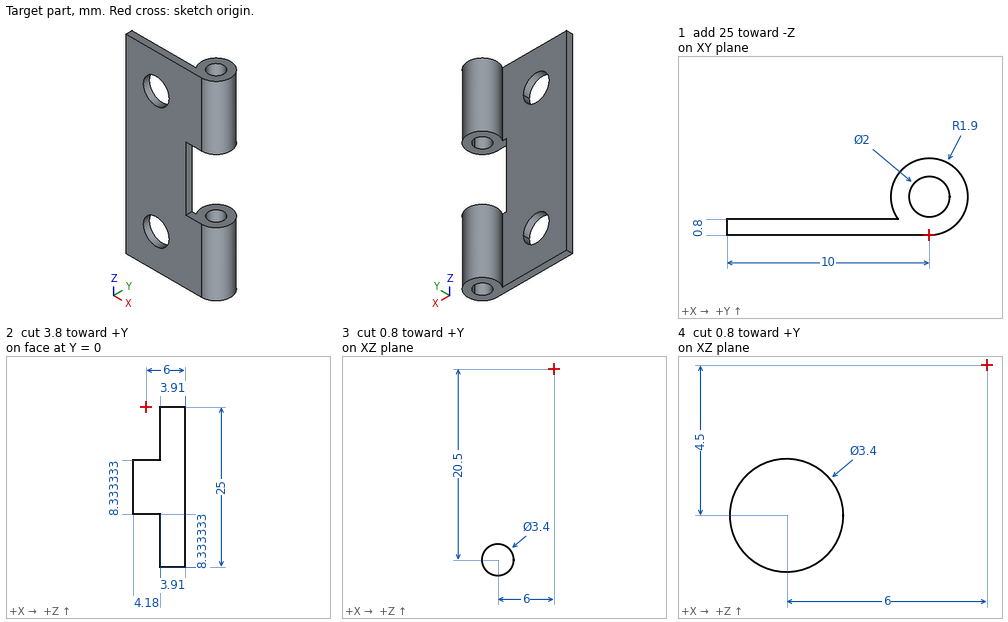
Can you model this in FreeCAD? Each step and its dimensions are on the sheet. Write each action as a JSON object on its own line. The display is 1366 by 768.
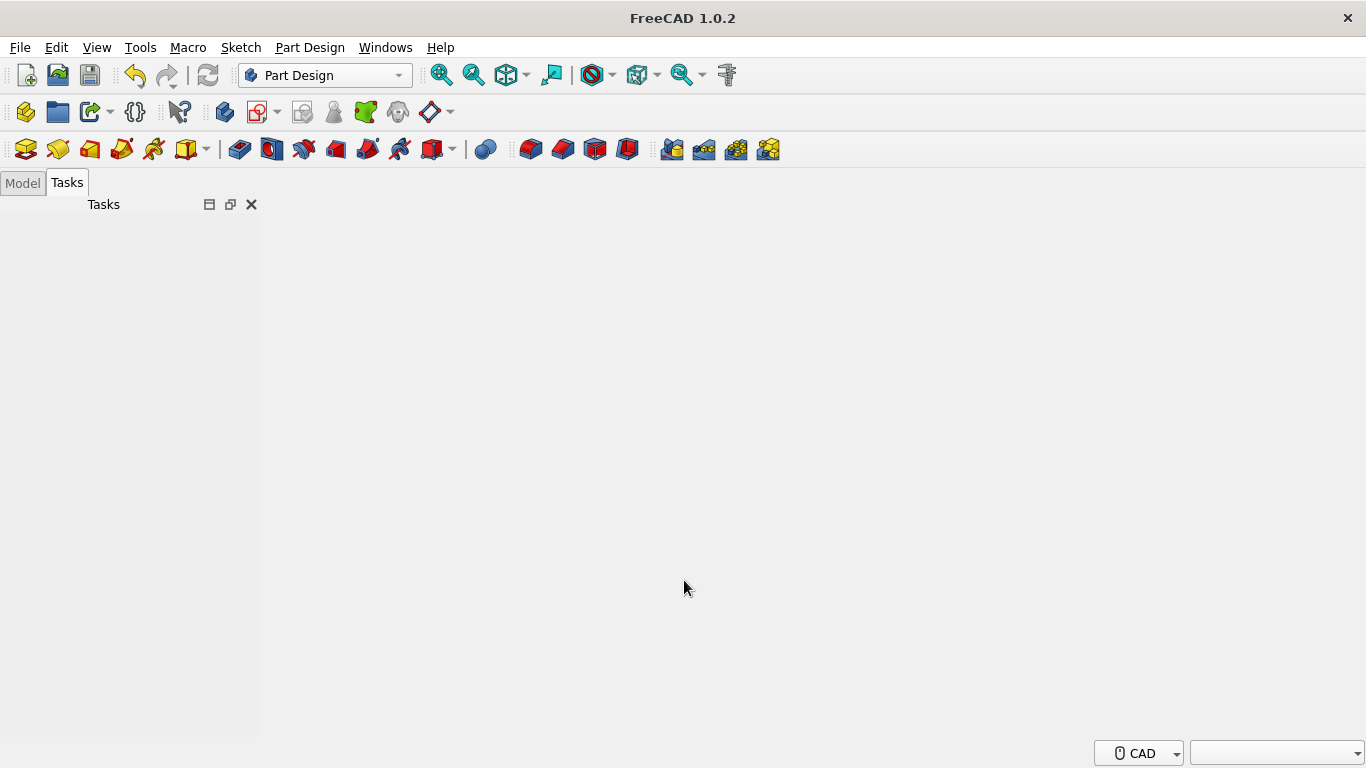
{"action": "left_click", "coordinate": [26, 76]}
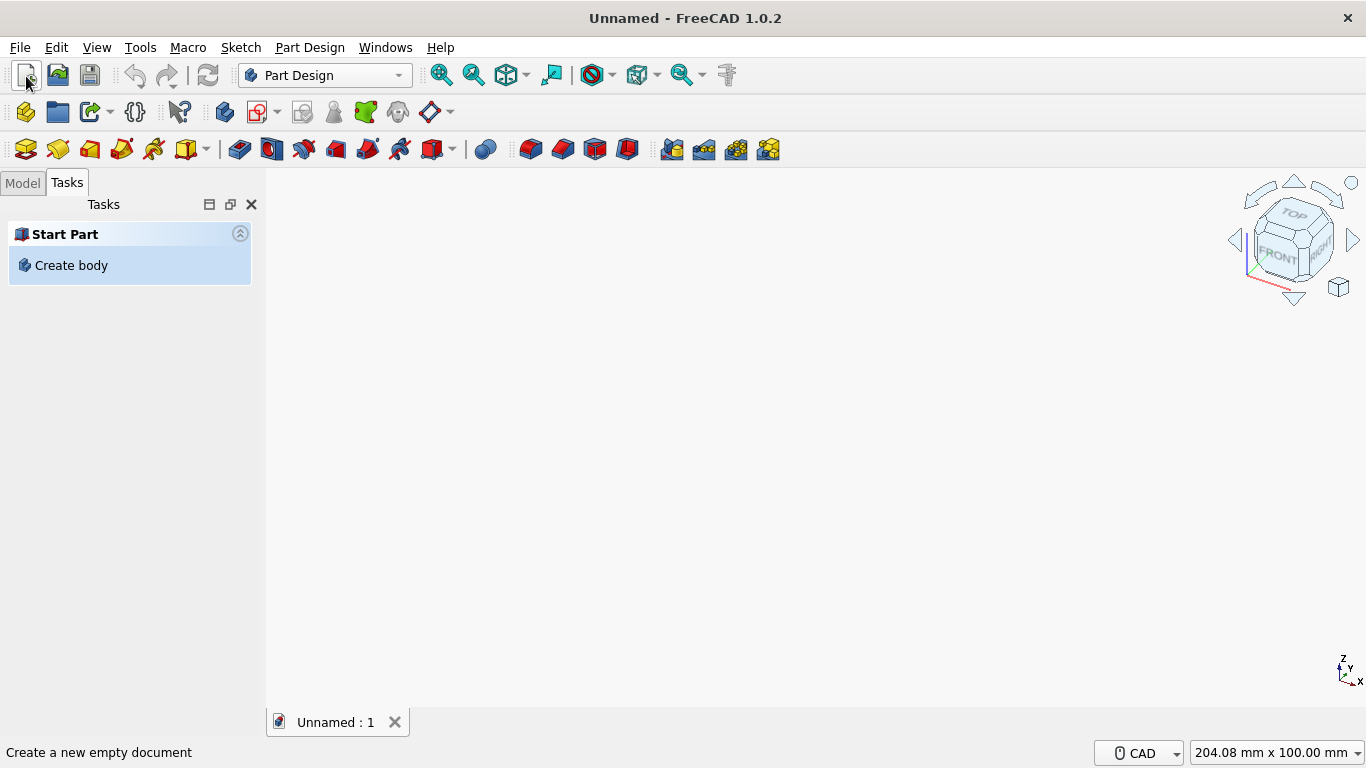
{"action": "left_click", "coordinate": [258, 112]}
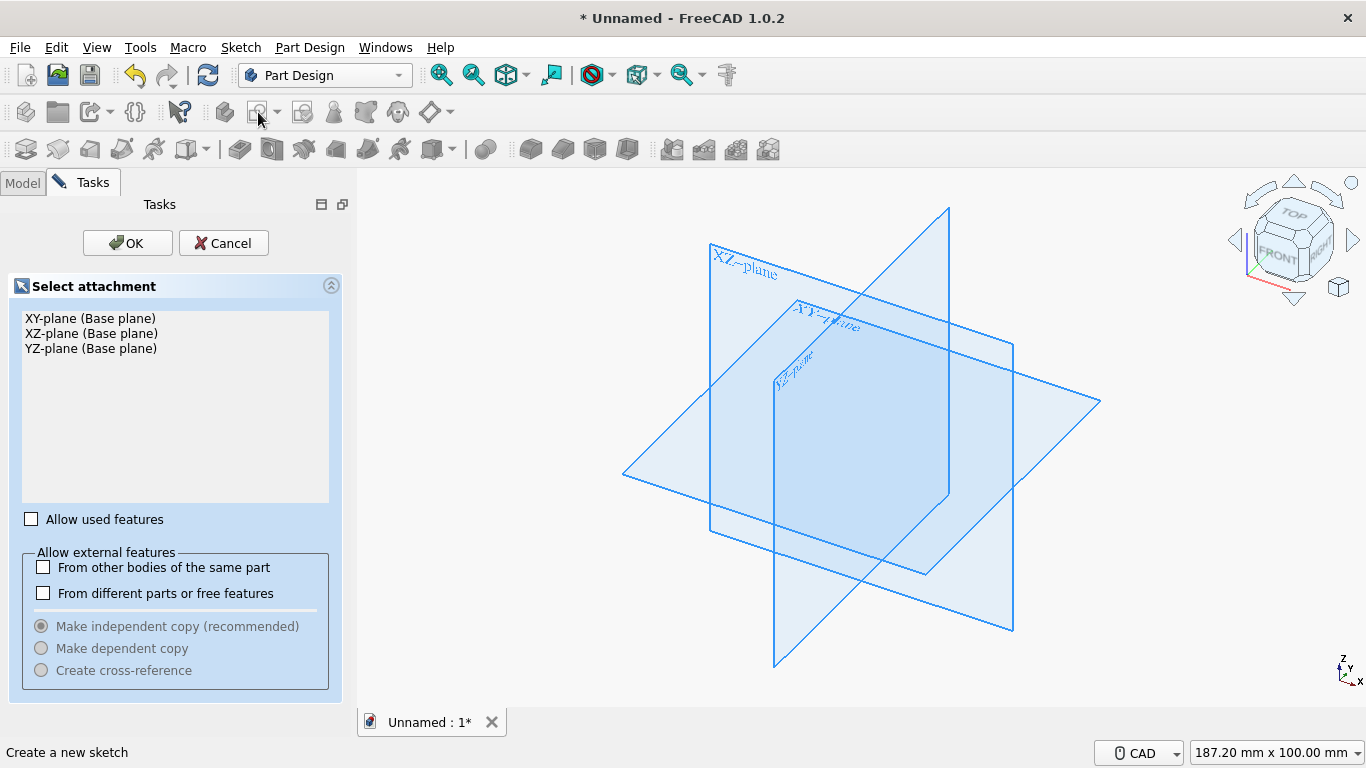
{"action": "left_click", "coordinate": [82, 318]}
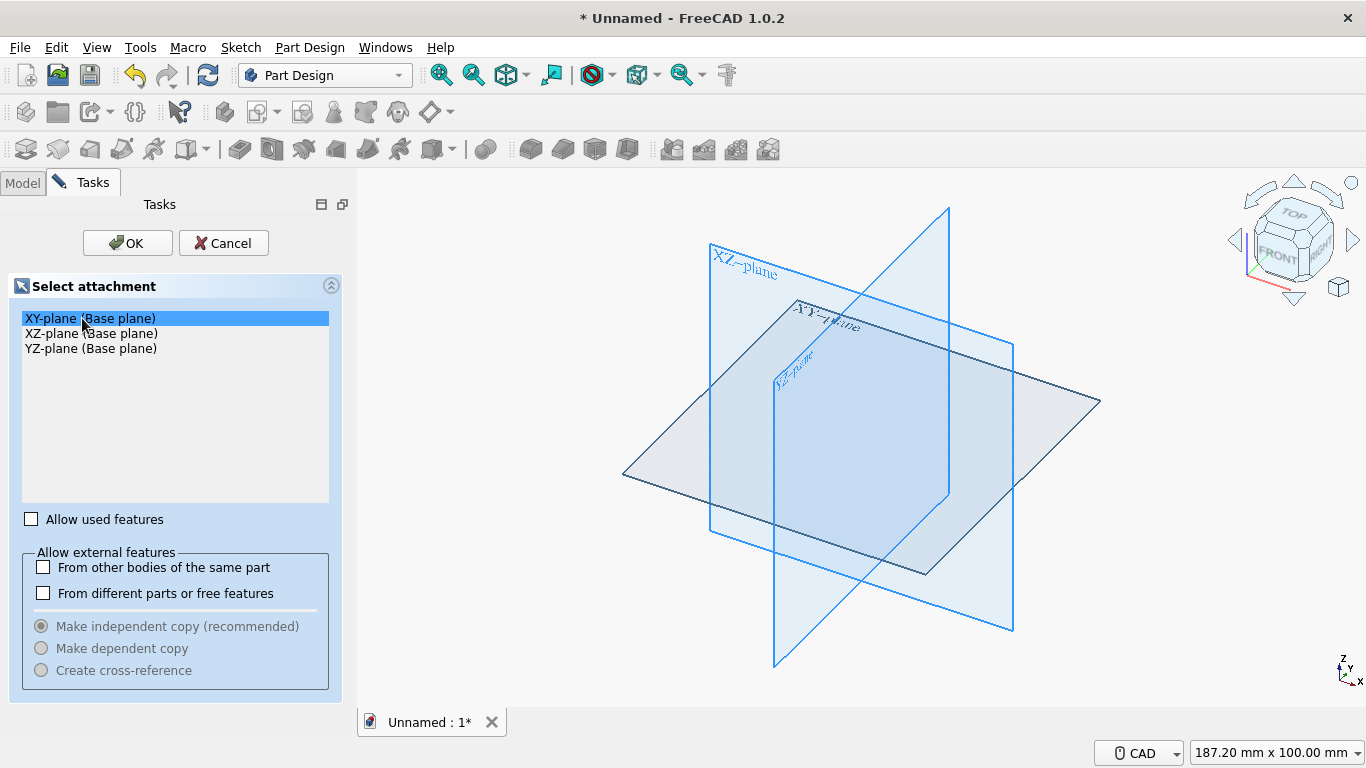
{"action": "left_click", "coordinate": [128, 243]}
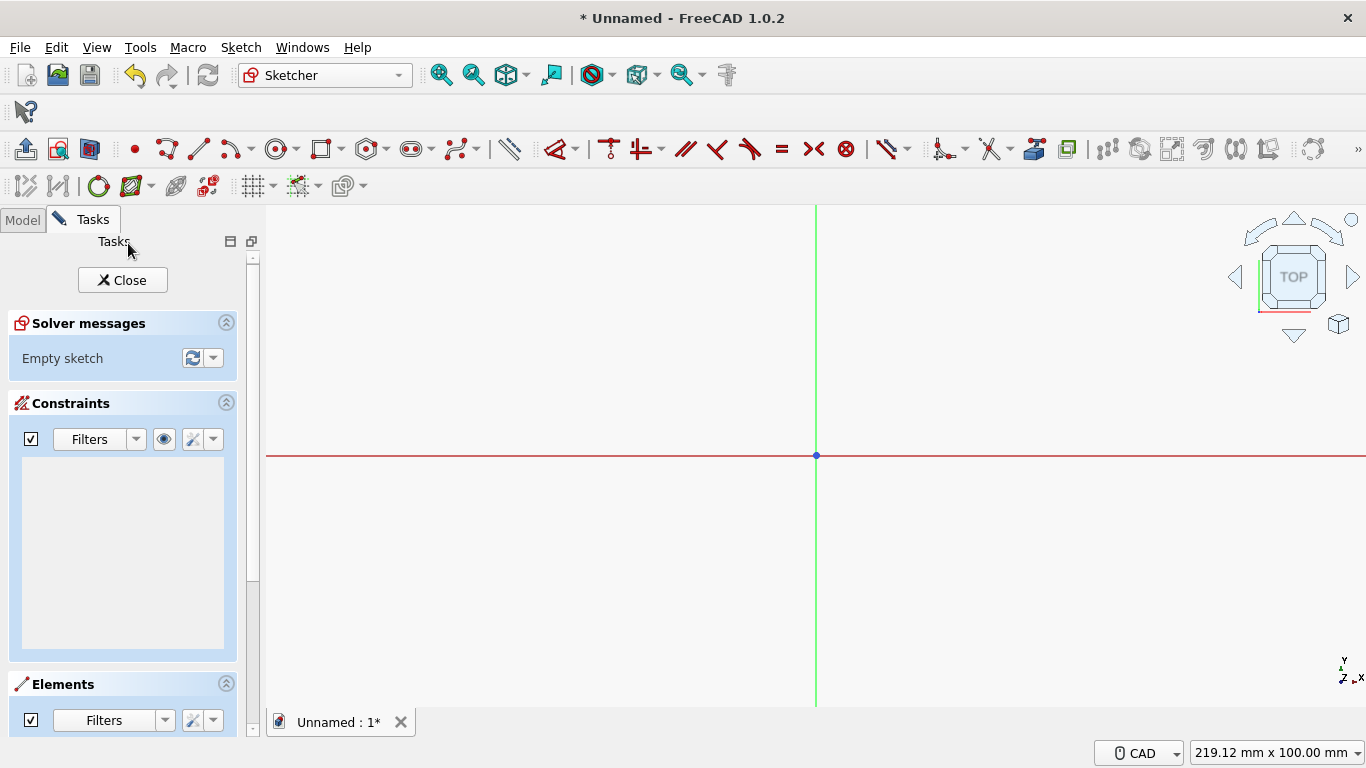
{"action": "scroll", "coordinate": [798, 446], "scroll_direction": "up", "scroll_amount": 12}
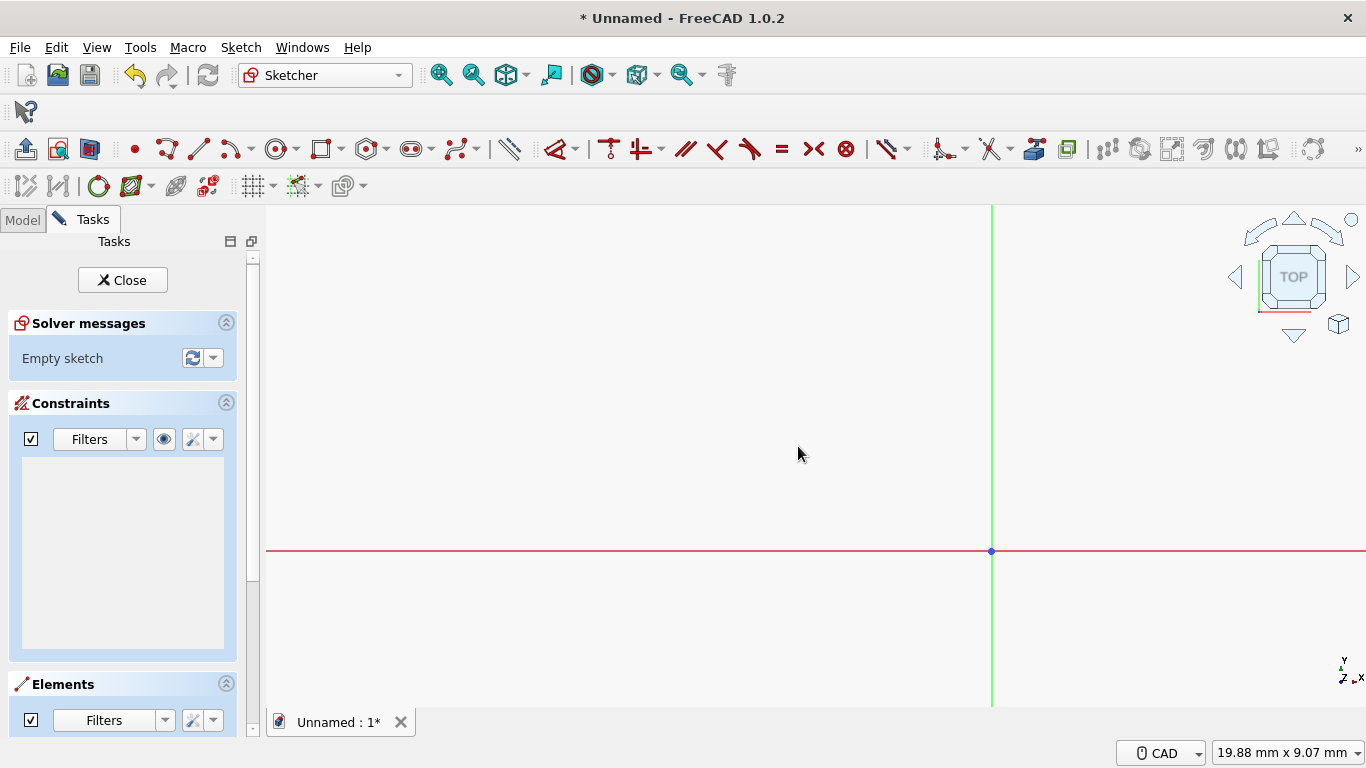
{"action": "left_click", "coordinate": [168, 150]}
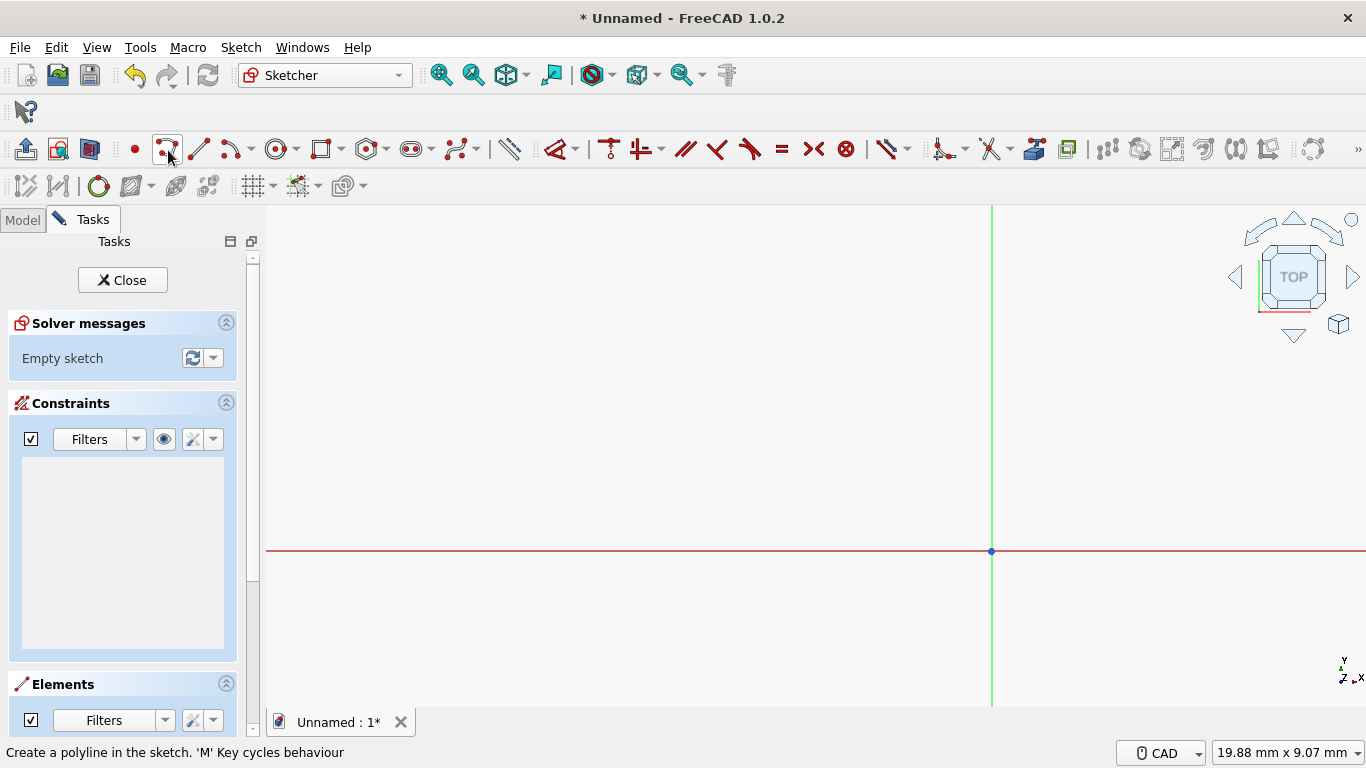
{"action": "left_click", "coordinate": [906, 507]}
{"action": "left_click", "coordinate": [438, 507]}
{"action": "left_click", "coordinate": [438, 551]}
{"action": "left_click", "coordinate": [992, 551]}
{"action": "right_click", "coordinate": [992, 551]}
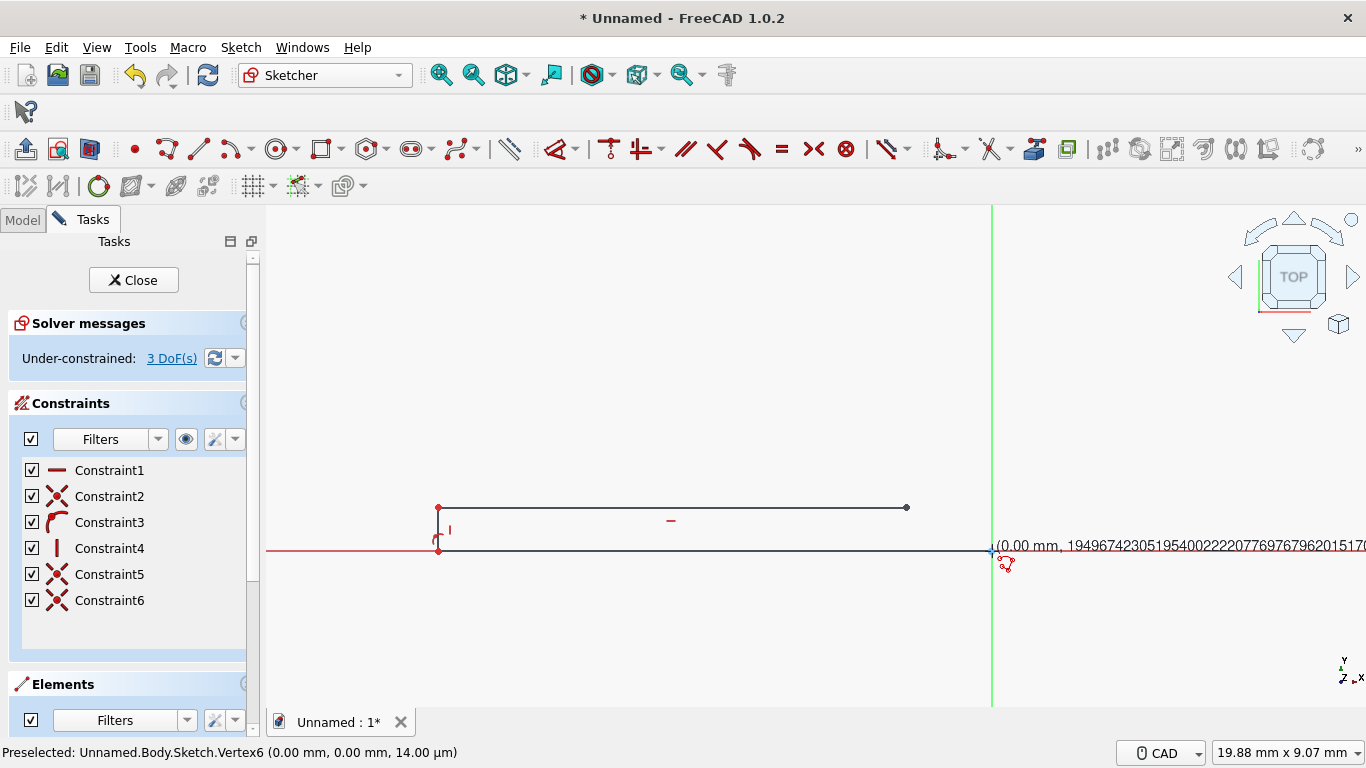
{"action": "key", "text": "g 3 a"}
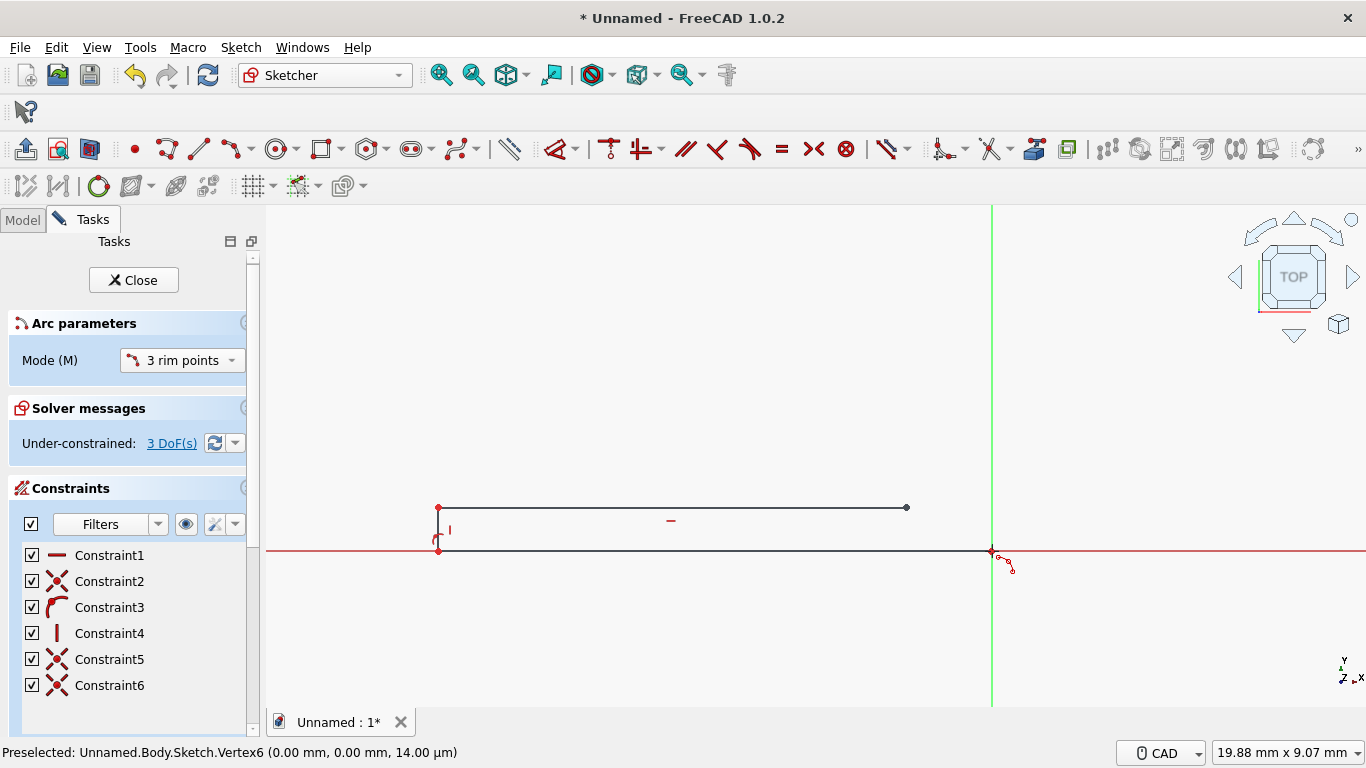
{"action": "left_click", "coordinate": [992, 551]}
{"action": "left_click", "coordinate": [906, 508]}
{"action": "left_click", "coordinate": [1040, 353]}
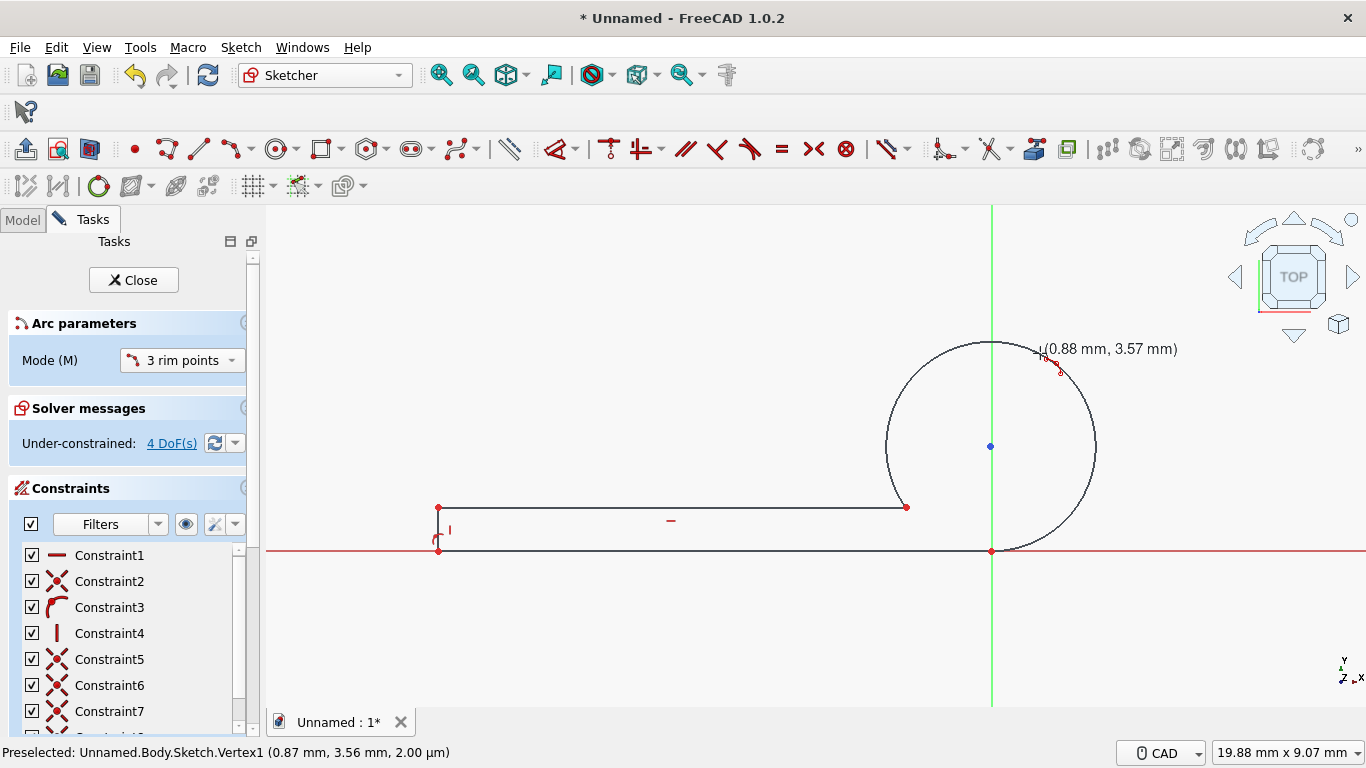
{"action": "left_click", "coordinate": [276, 150]}